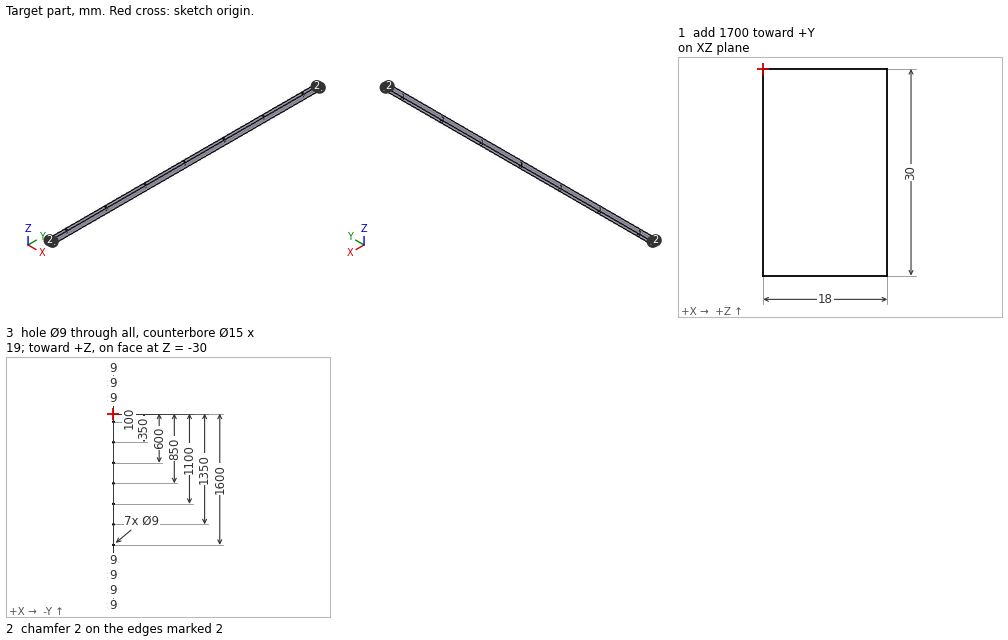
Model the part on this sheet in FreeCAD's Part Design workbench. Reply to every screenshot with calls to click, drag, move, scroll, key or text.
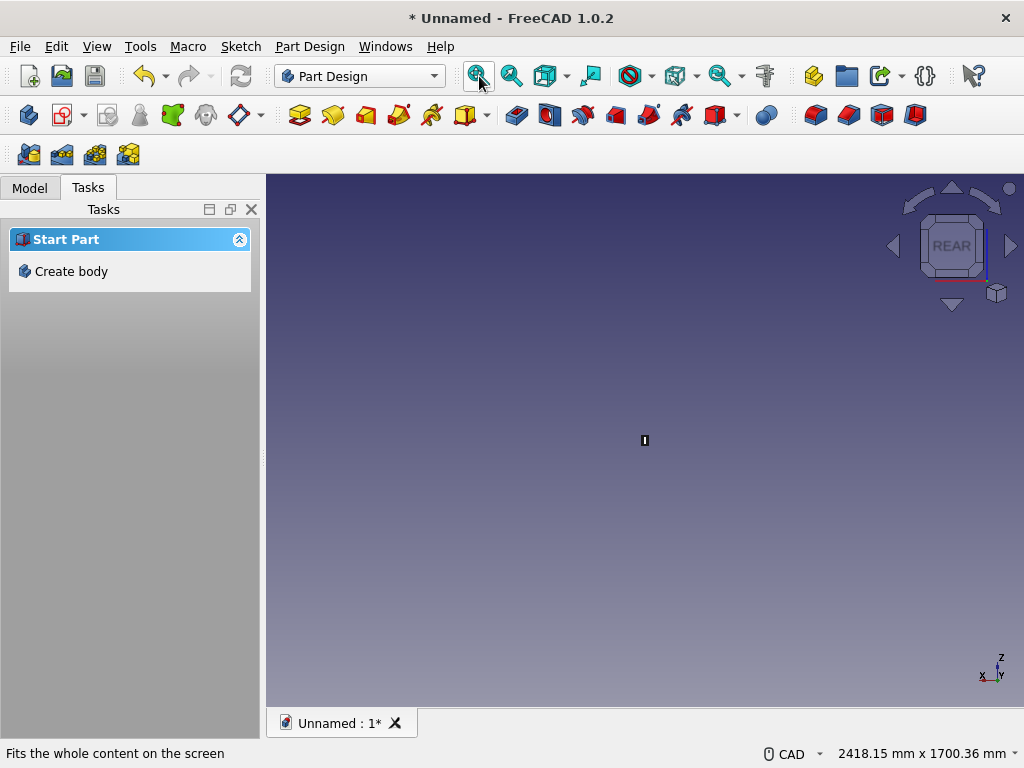
key(5)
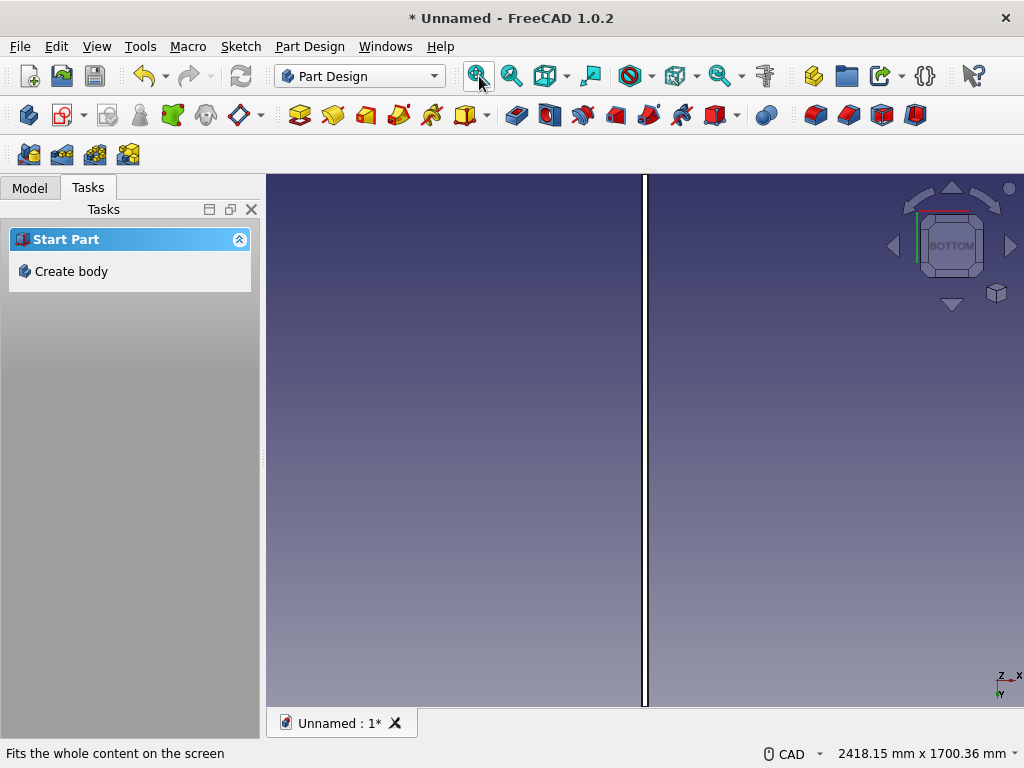
key(v)
key(f)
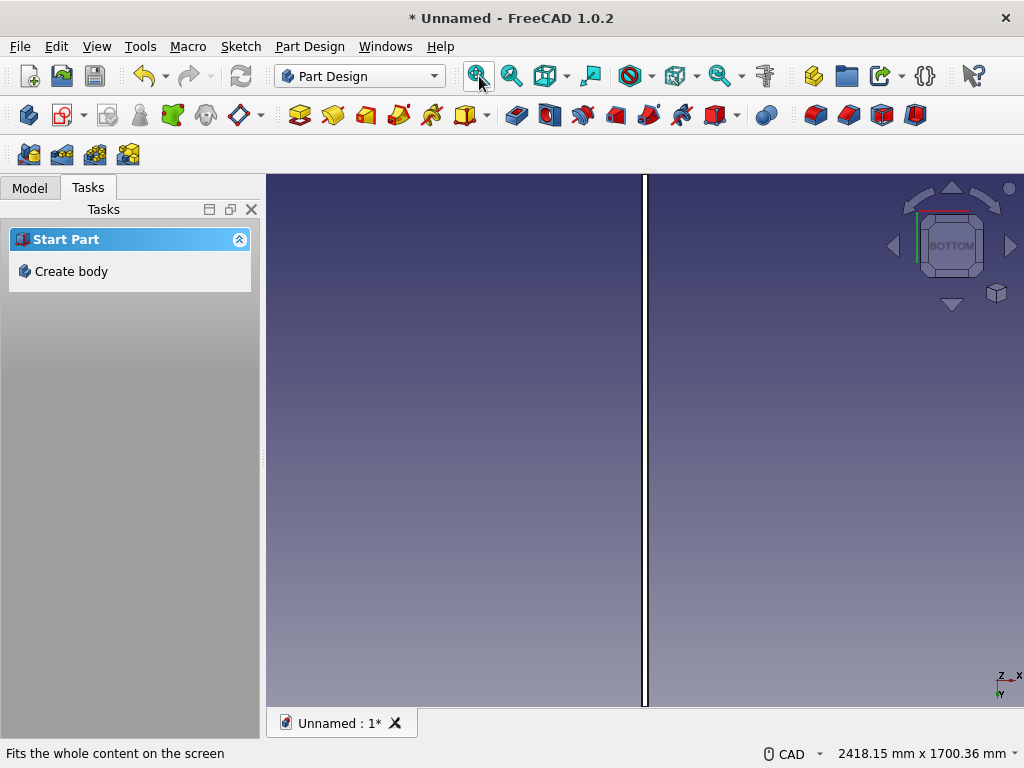
scroll(645, 668, up, 8)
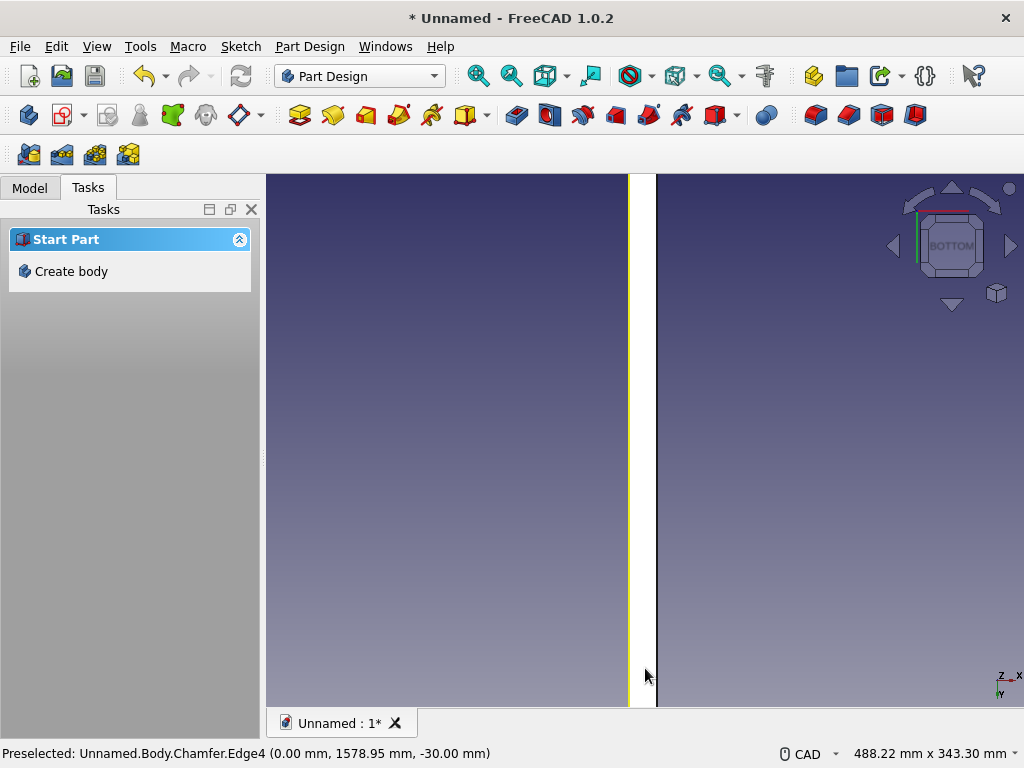
click(643, 668)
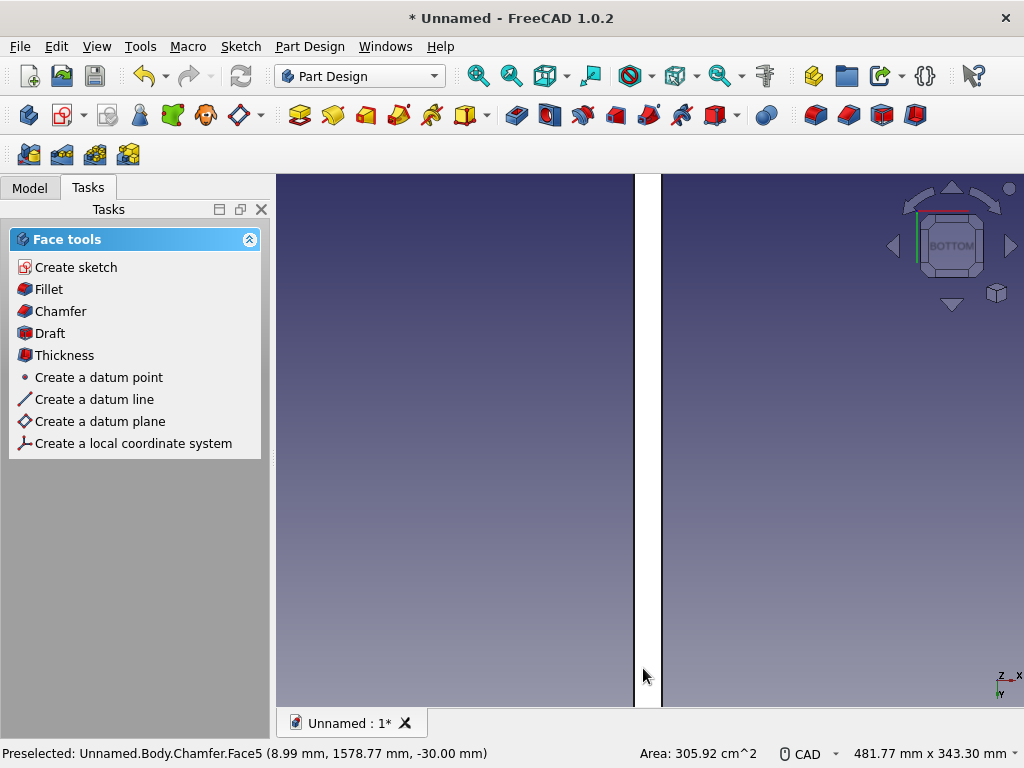
click(62, 116)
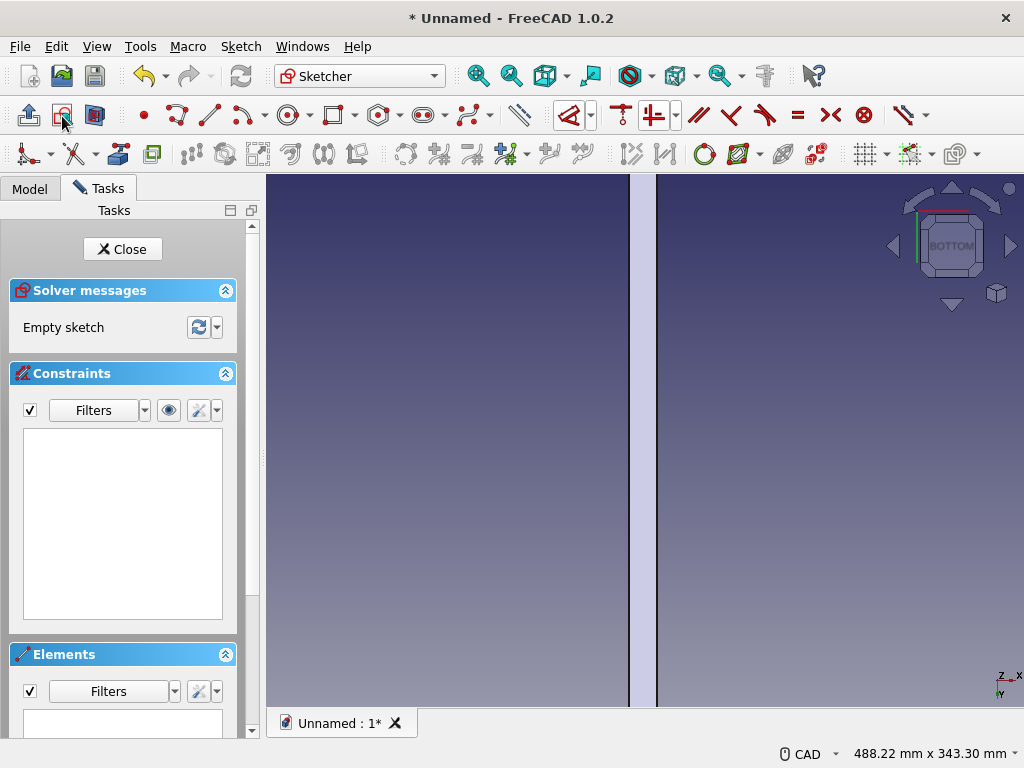
scroll(567, 593, down, 10)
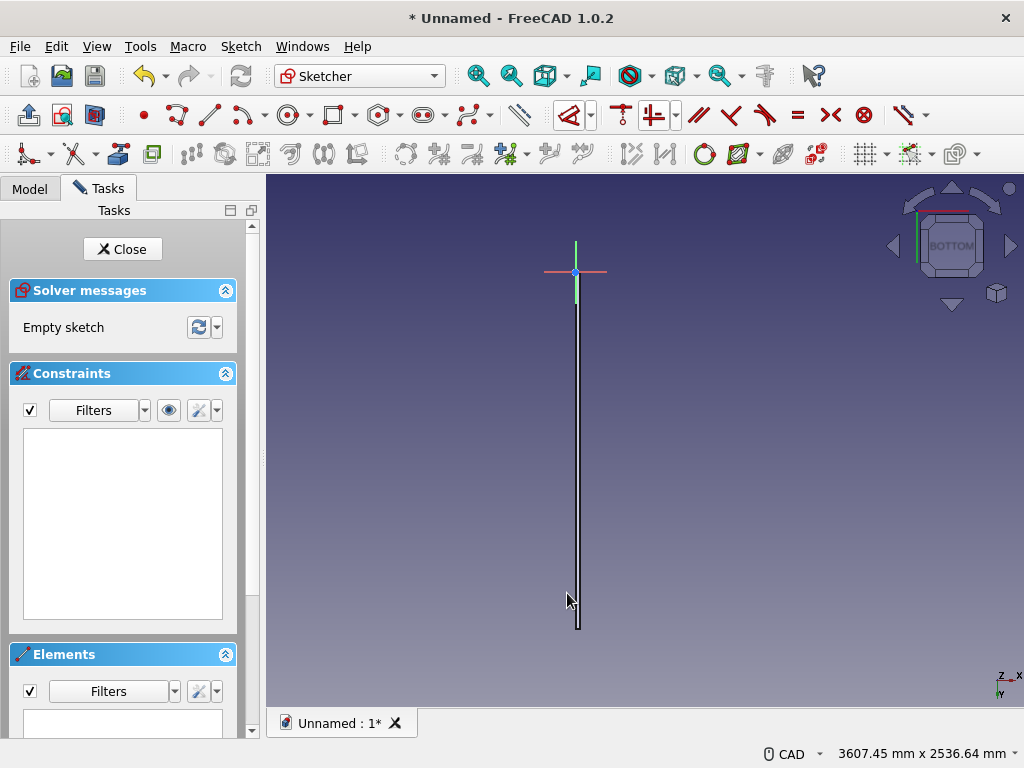
click(288, 116)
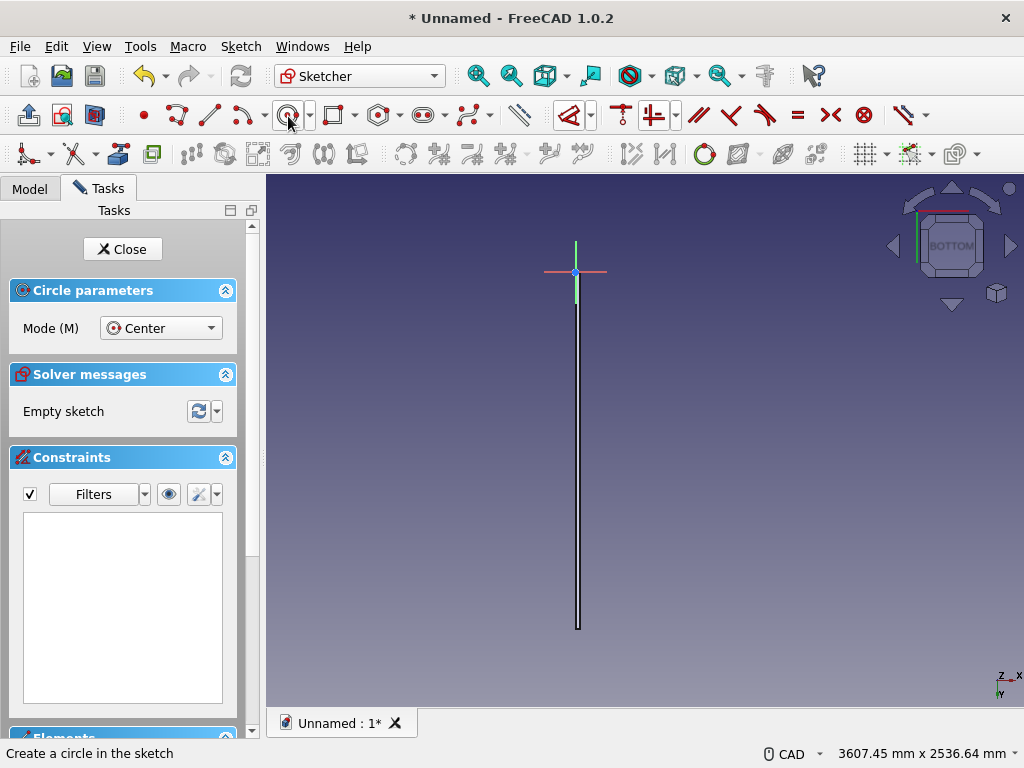
scroll(578, 608, up, 16)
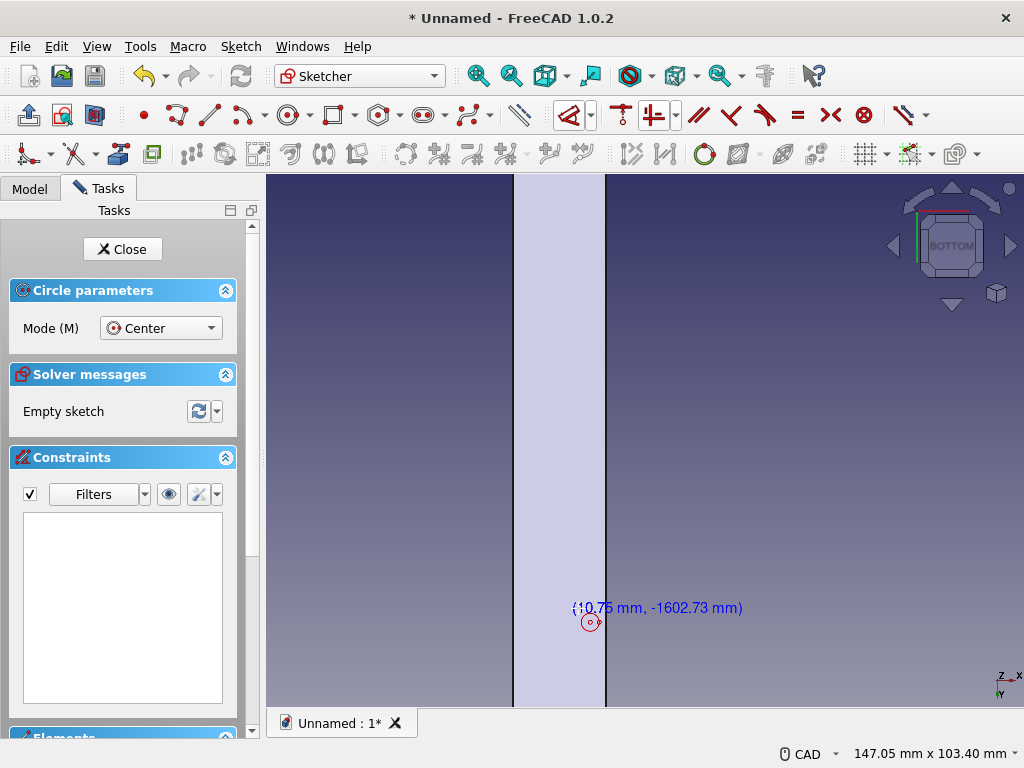
scroll(578, 648, down, 15)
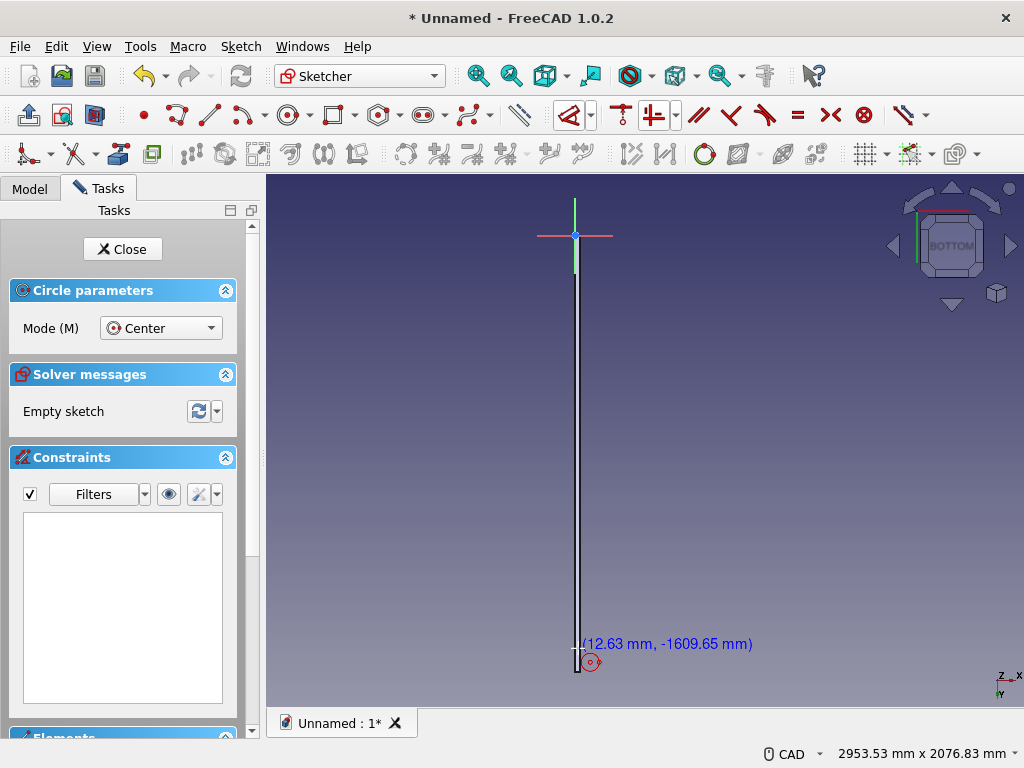
scroll(577, 646, up, 10)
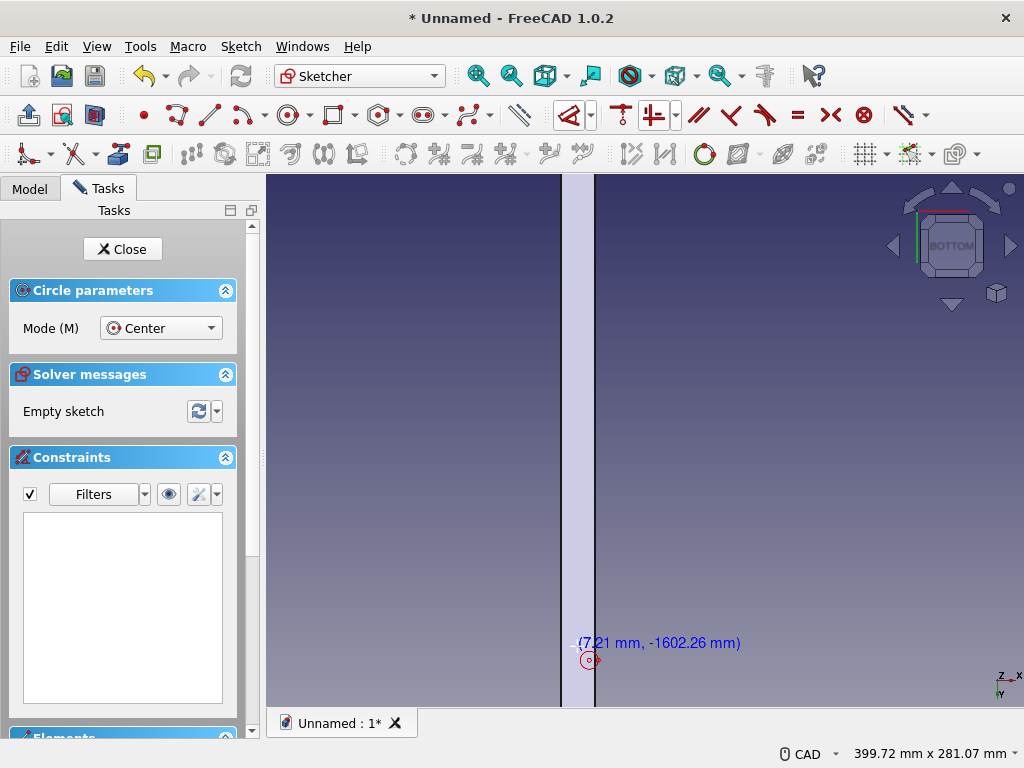
click(578, 643)
move(584, 637)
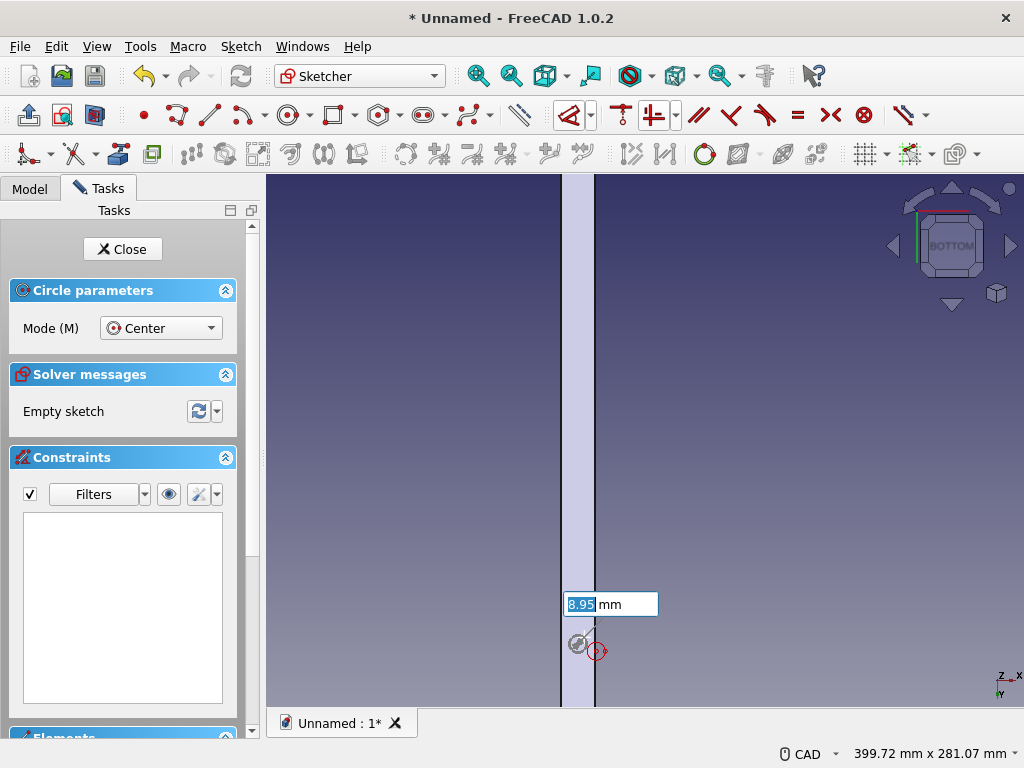
text(9)
key(Return)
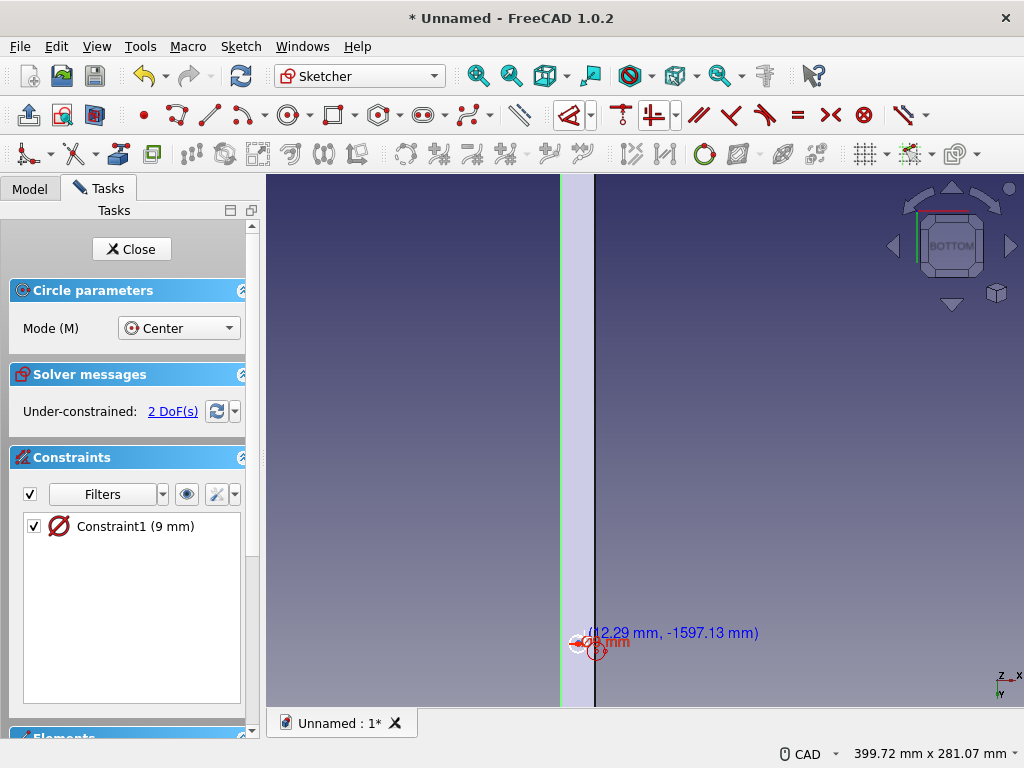
scroll(577, 604, down, 11)